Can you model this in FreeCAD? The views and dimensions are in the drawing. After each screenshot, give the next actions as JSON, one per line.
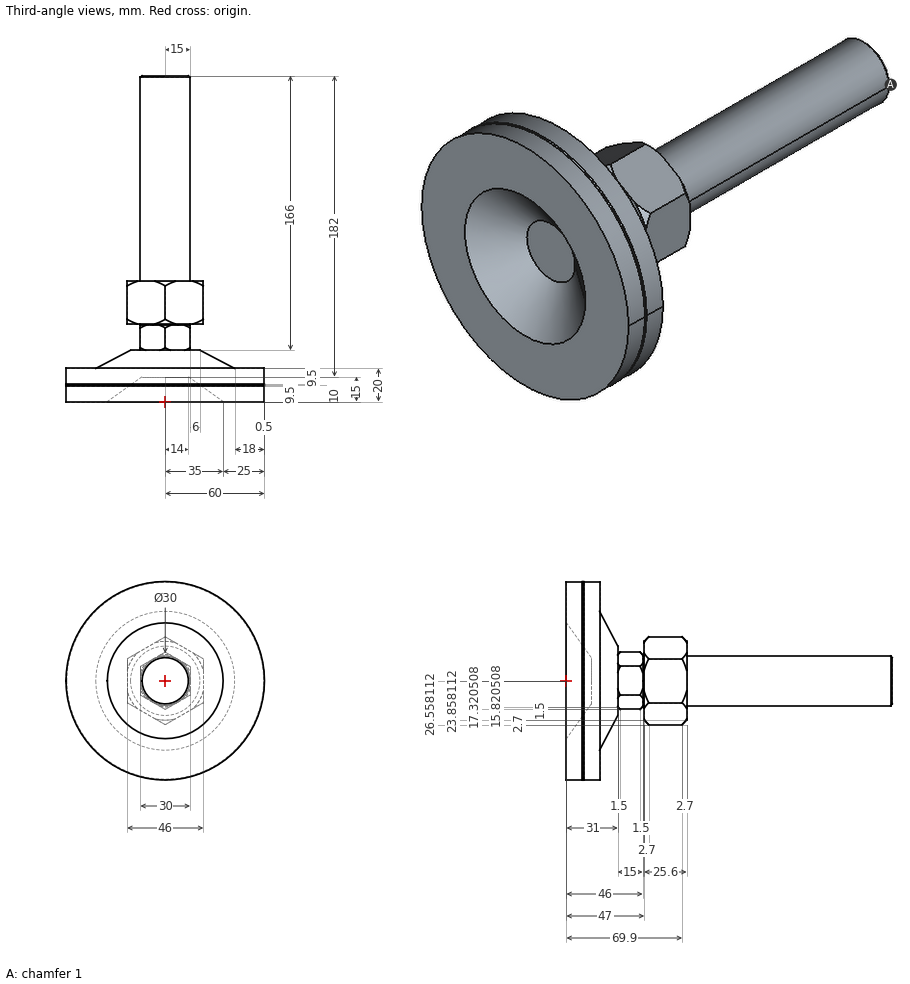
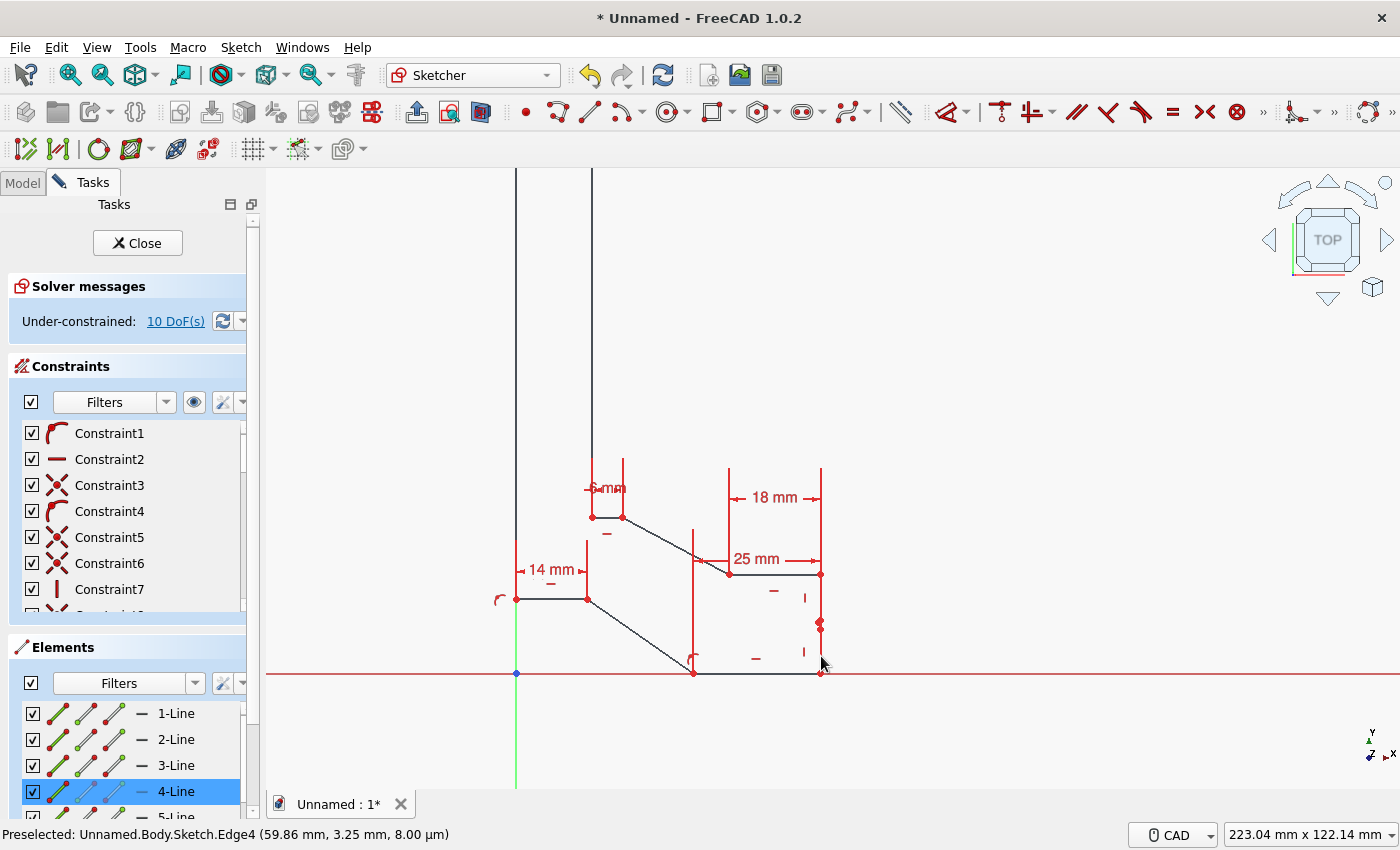
{"action": "left_click", "coordinate": [968, 112]}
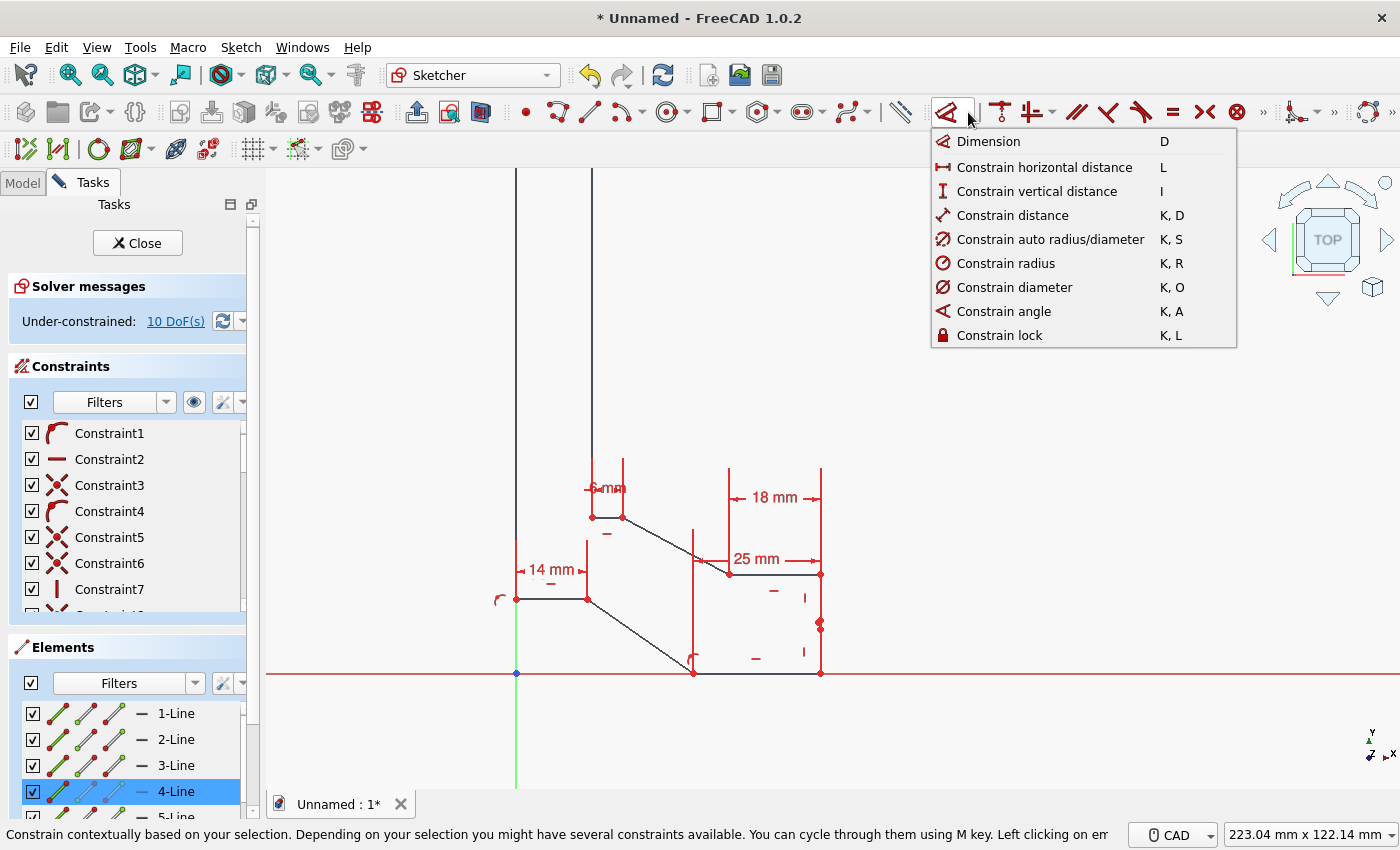
{"action": "left_click", "coordinate": [1084, 191]}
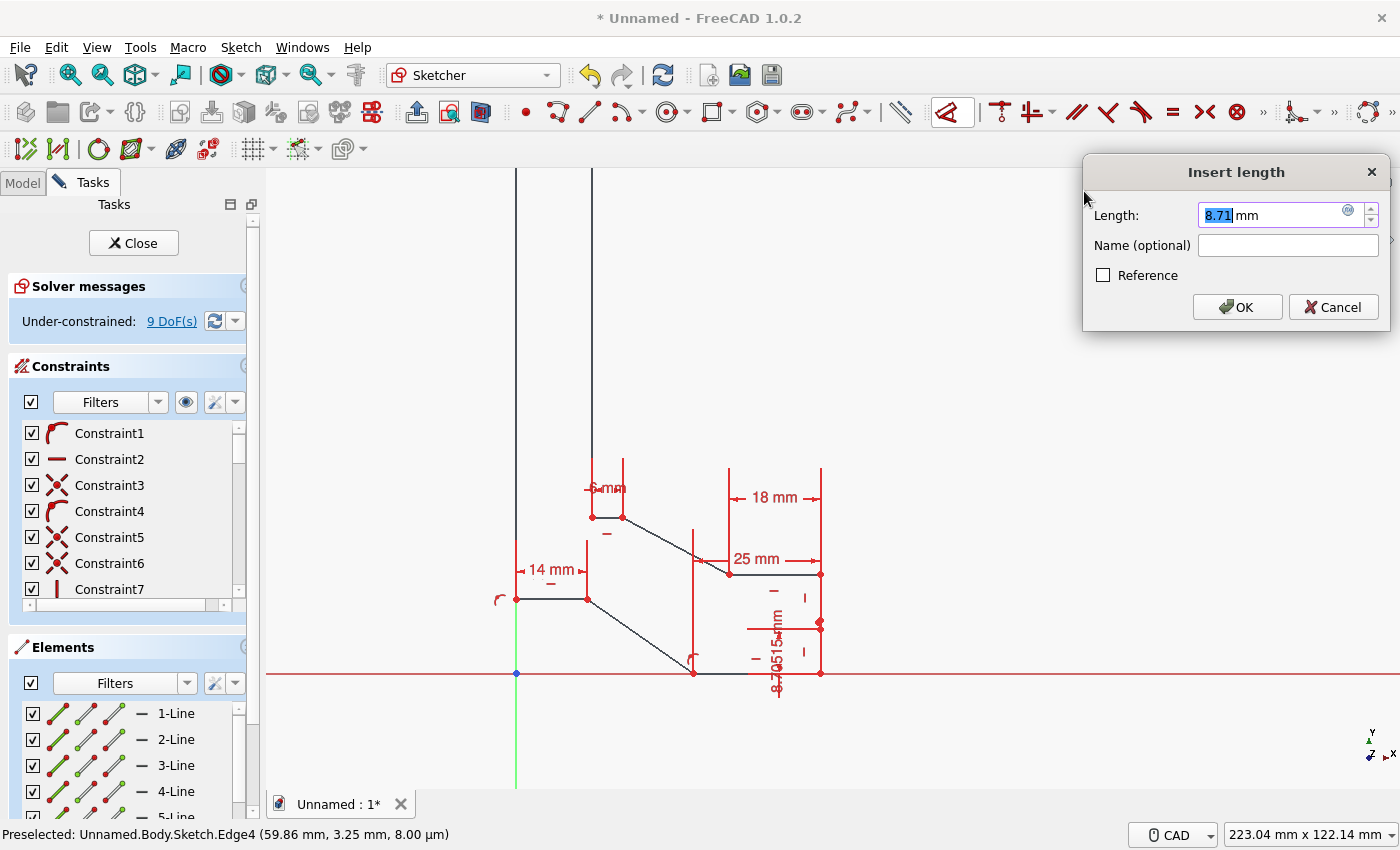
{"action": "type", "text": "9.5"}
{"action": "key", "text": "Return"}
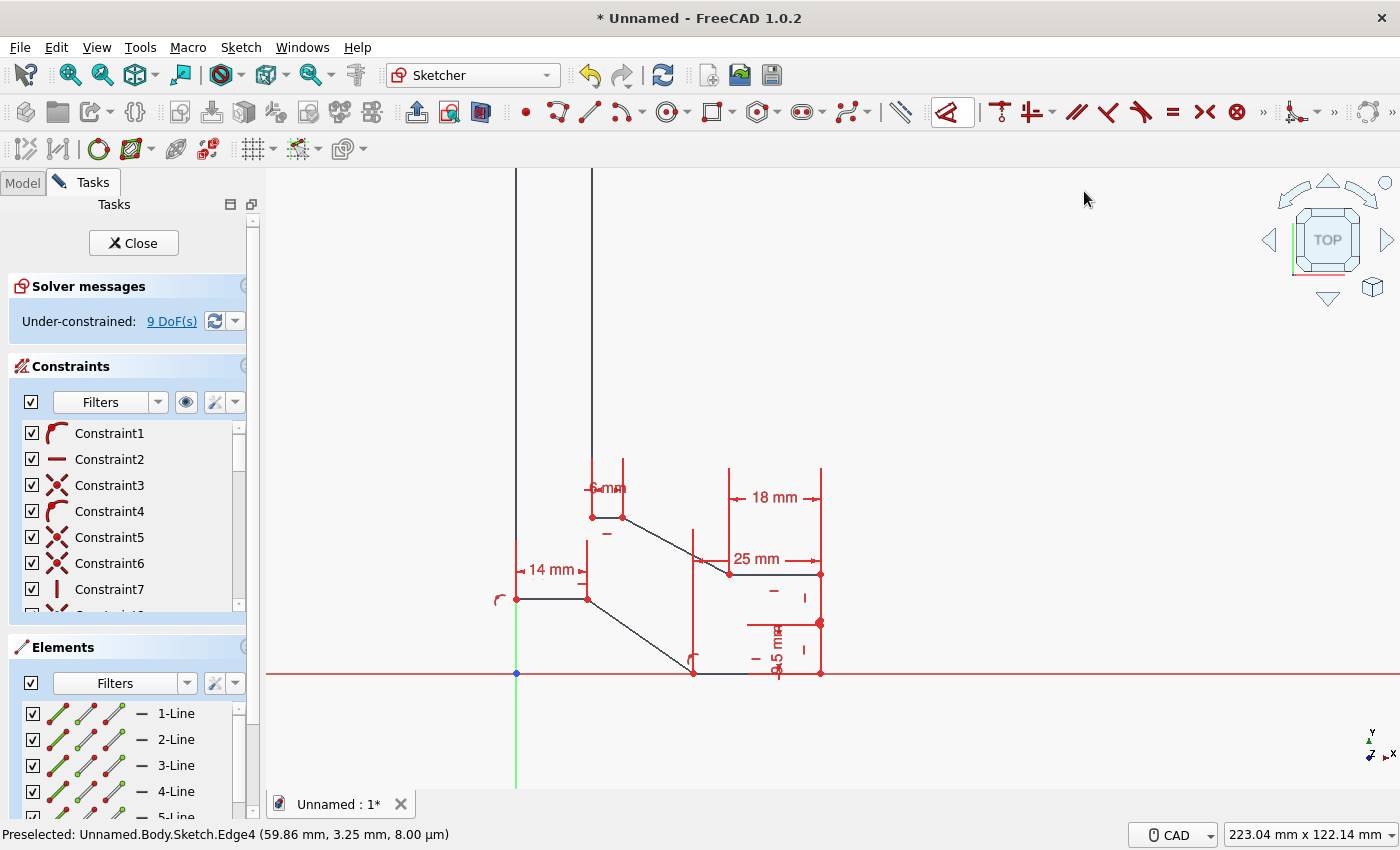
{"action": "left_click", "coordinate": [821, 607]}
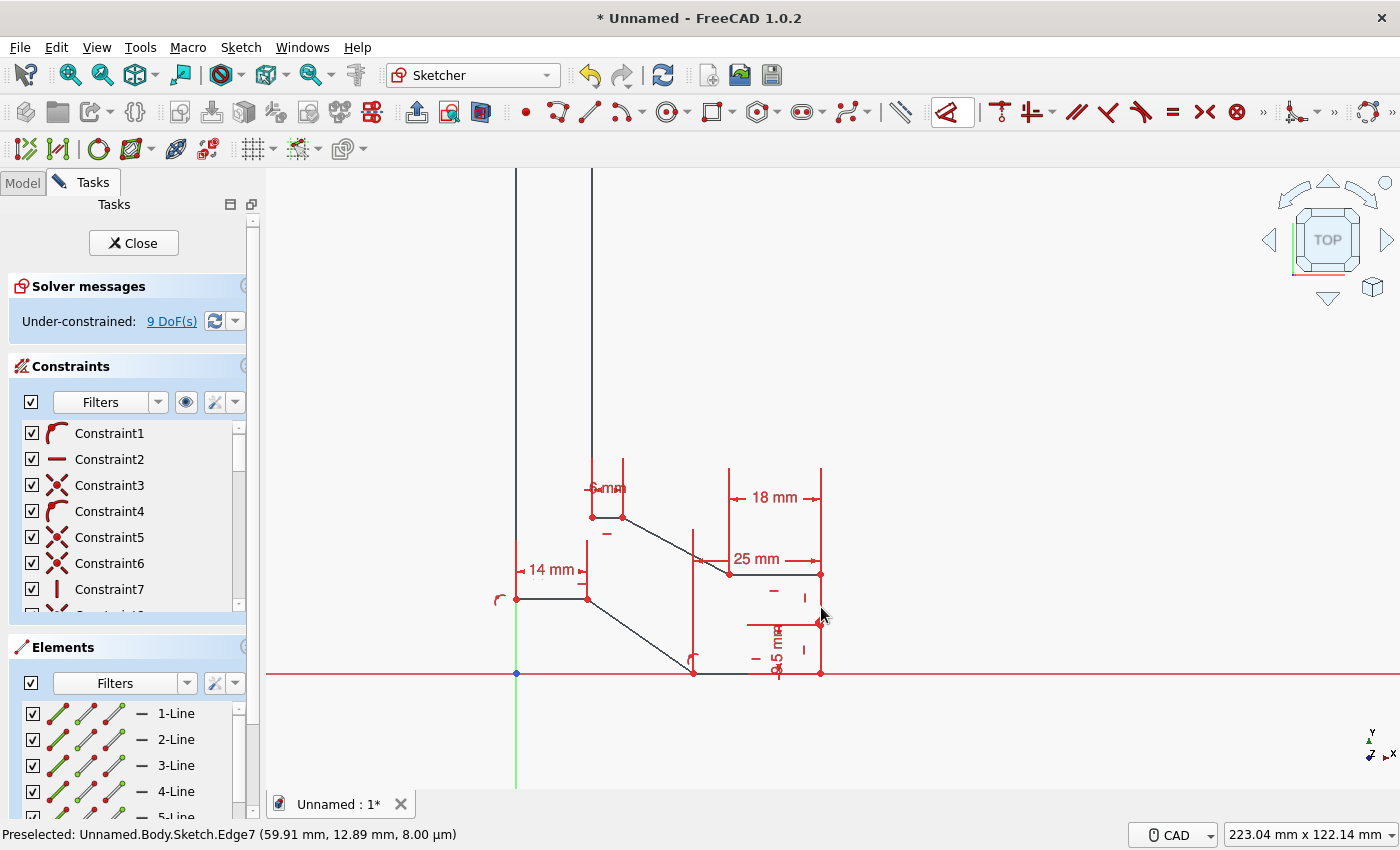
{"action": "key", "text": "i"}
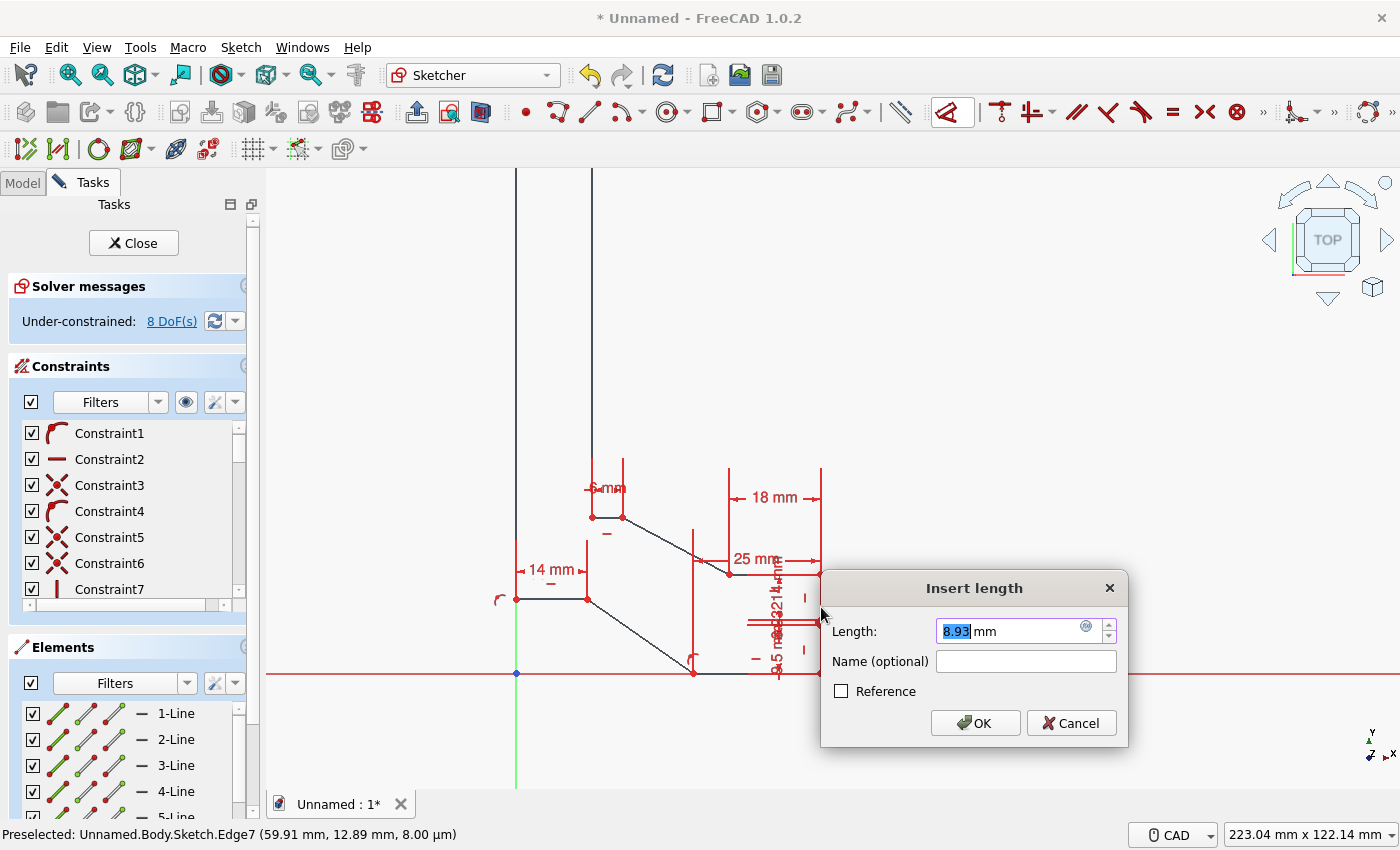
{"action": "type", "text": "9.5"}
{"action": "key", "text": "Return"}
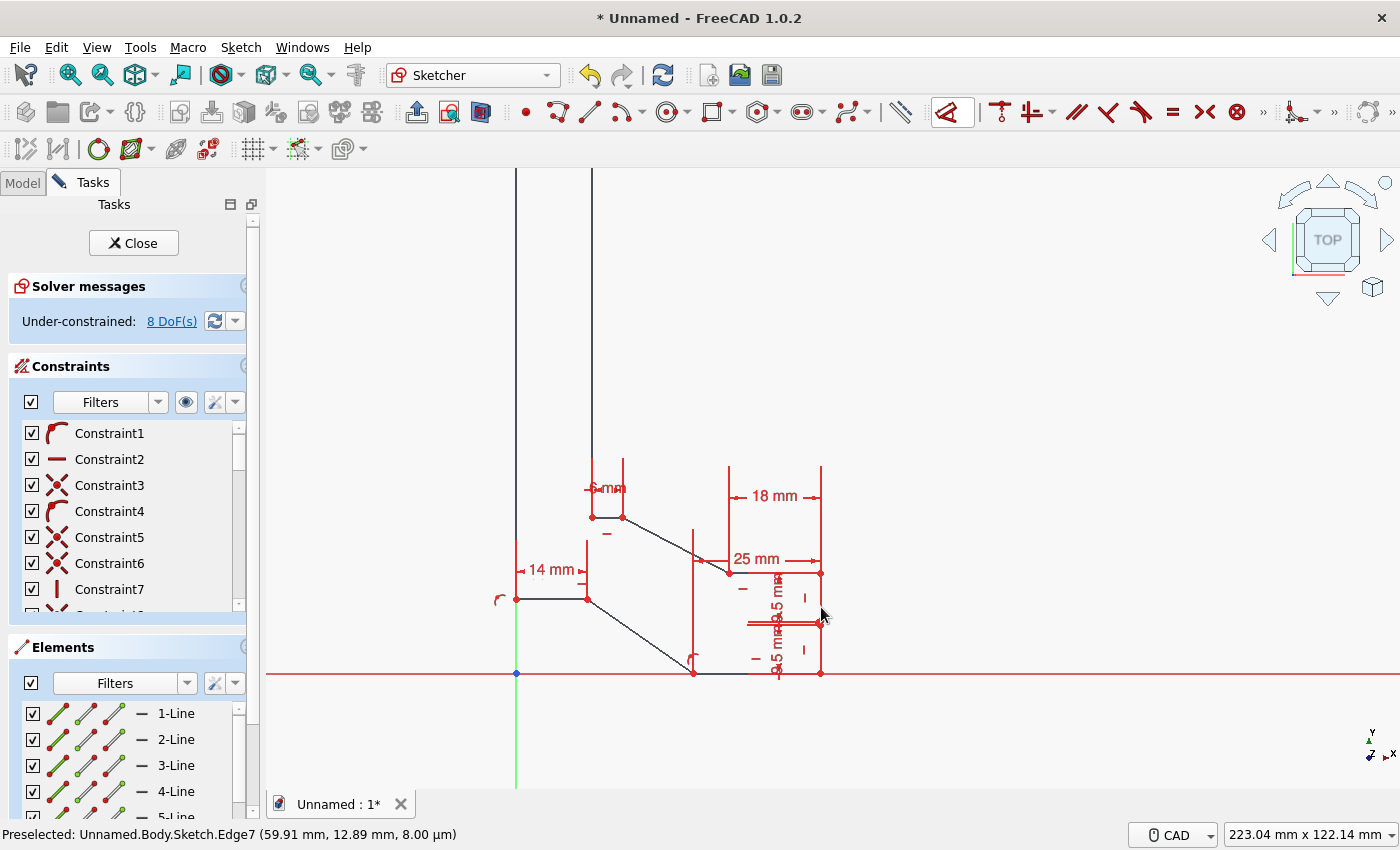
{"action": "left_click", "coordinate": [592, 264]}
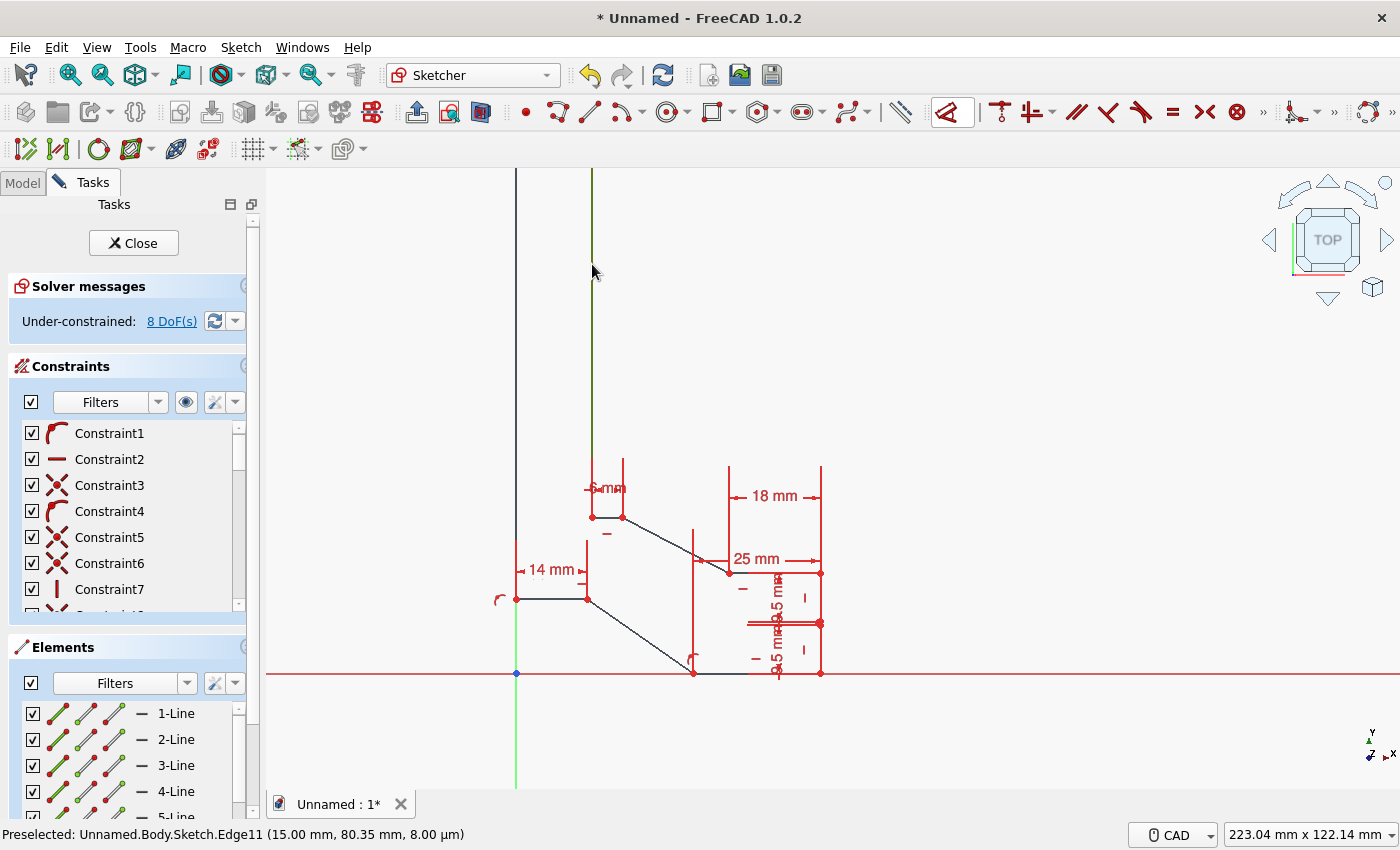
{"action": "left_click", "coordinate": [968, 112]}